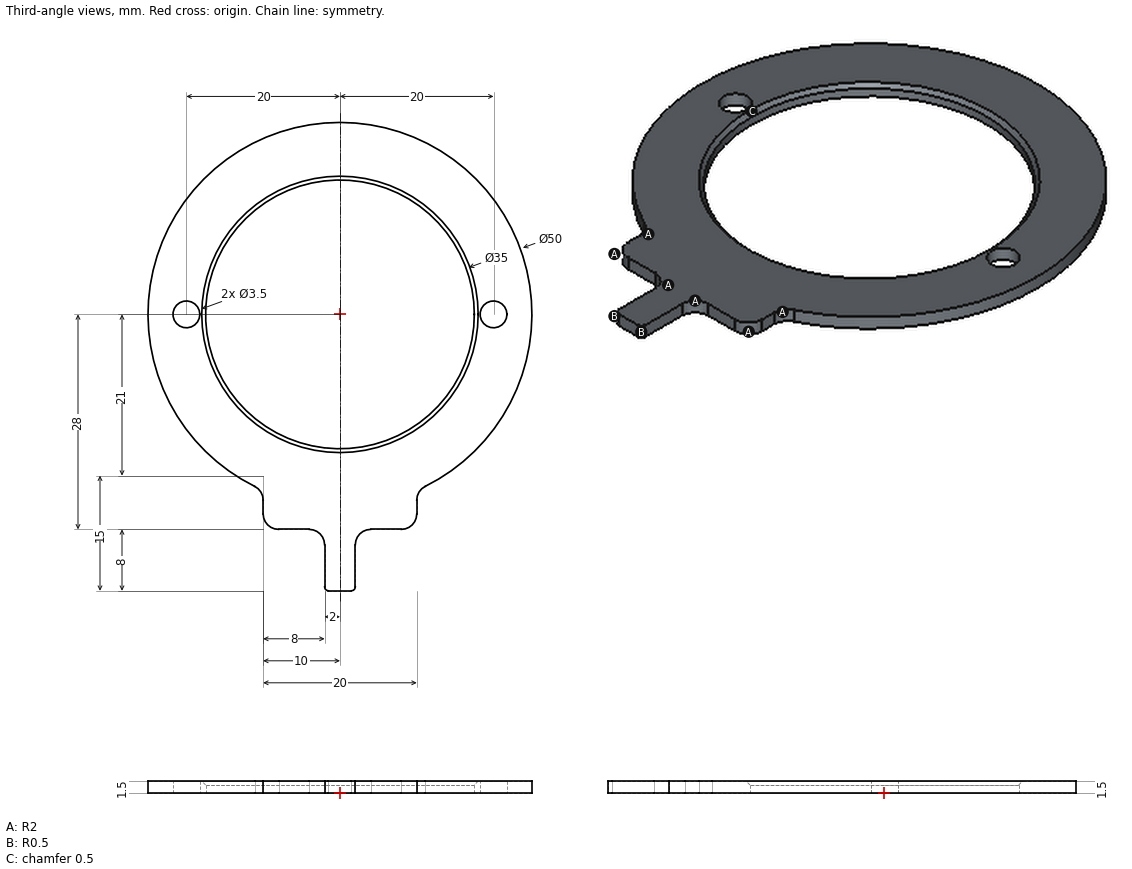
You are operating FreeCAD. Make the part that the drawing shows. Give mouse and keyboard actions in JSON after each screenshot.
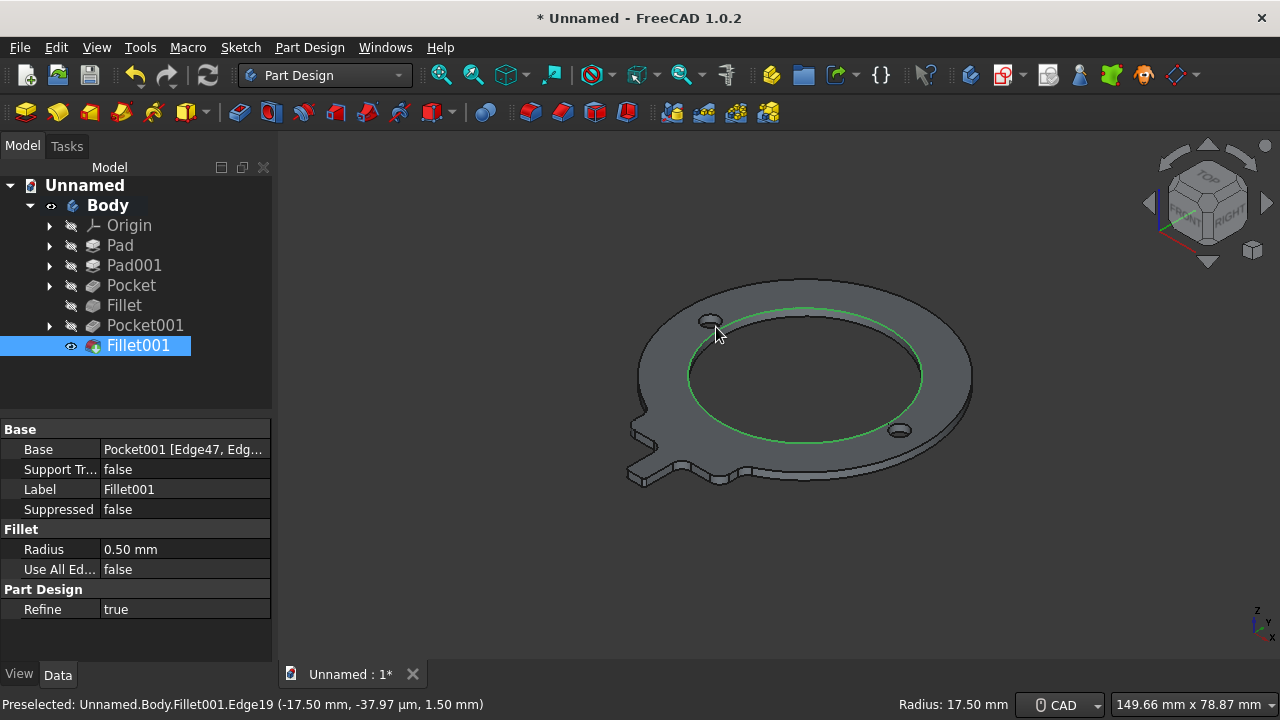
{"action": "left_click", "coordinate": [564, 112]}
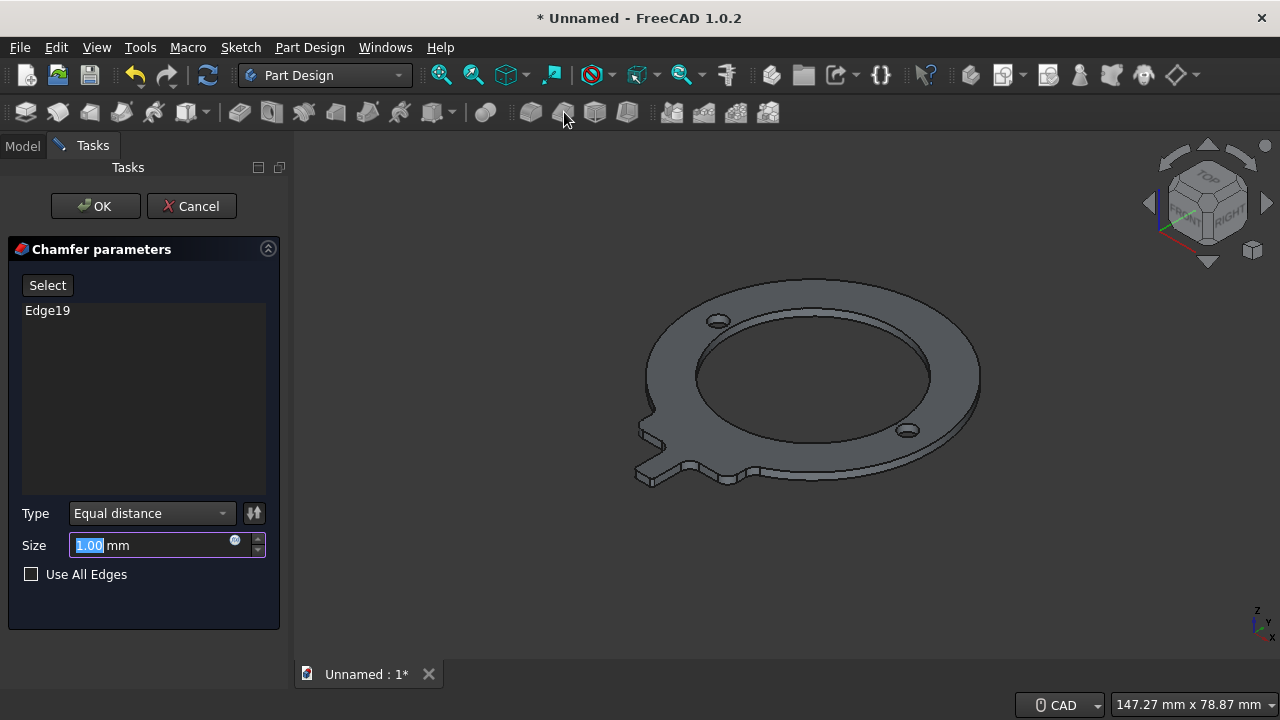
{"action": "type", "text": "0.5"}
{"action": "key", "text": "Tab"}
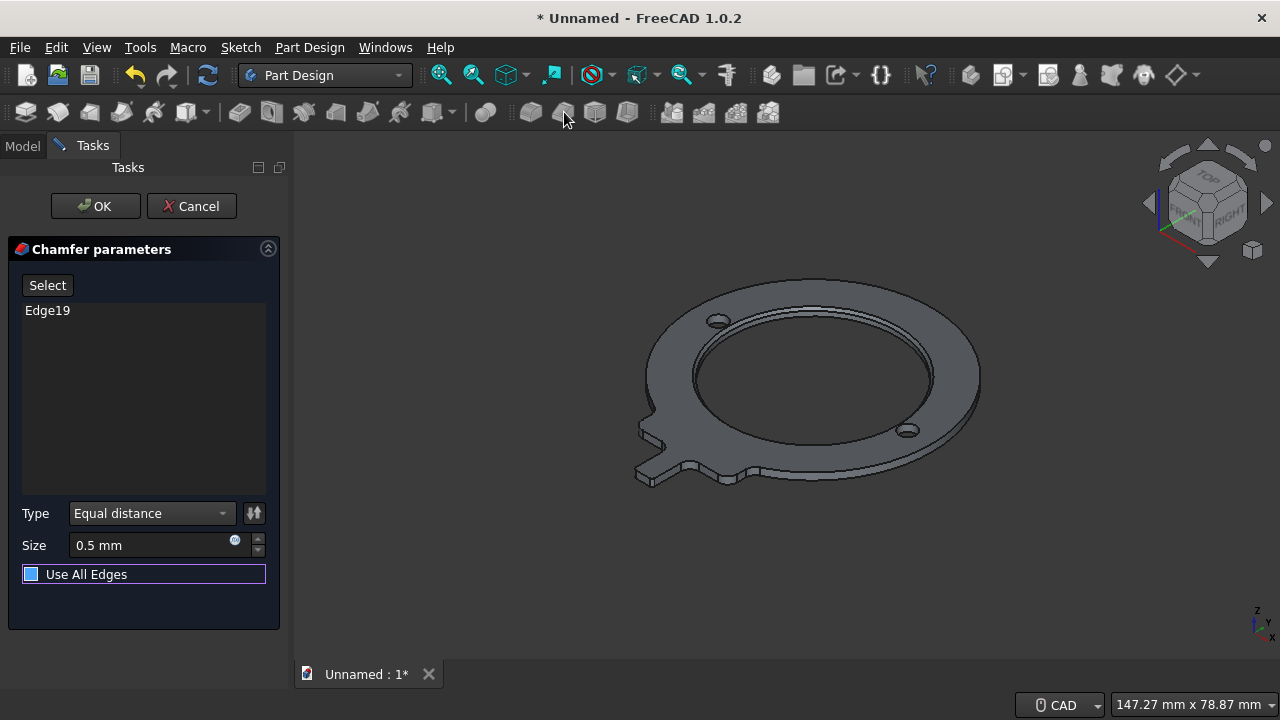
{"action": "left_click", "coordinate": [96, 206]}